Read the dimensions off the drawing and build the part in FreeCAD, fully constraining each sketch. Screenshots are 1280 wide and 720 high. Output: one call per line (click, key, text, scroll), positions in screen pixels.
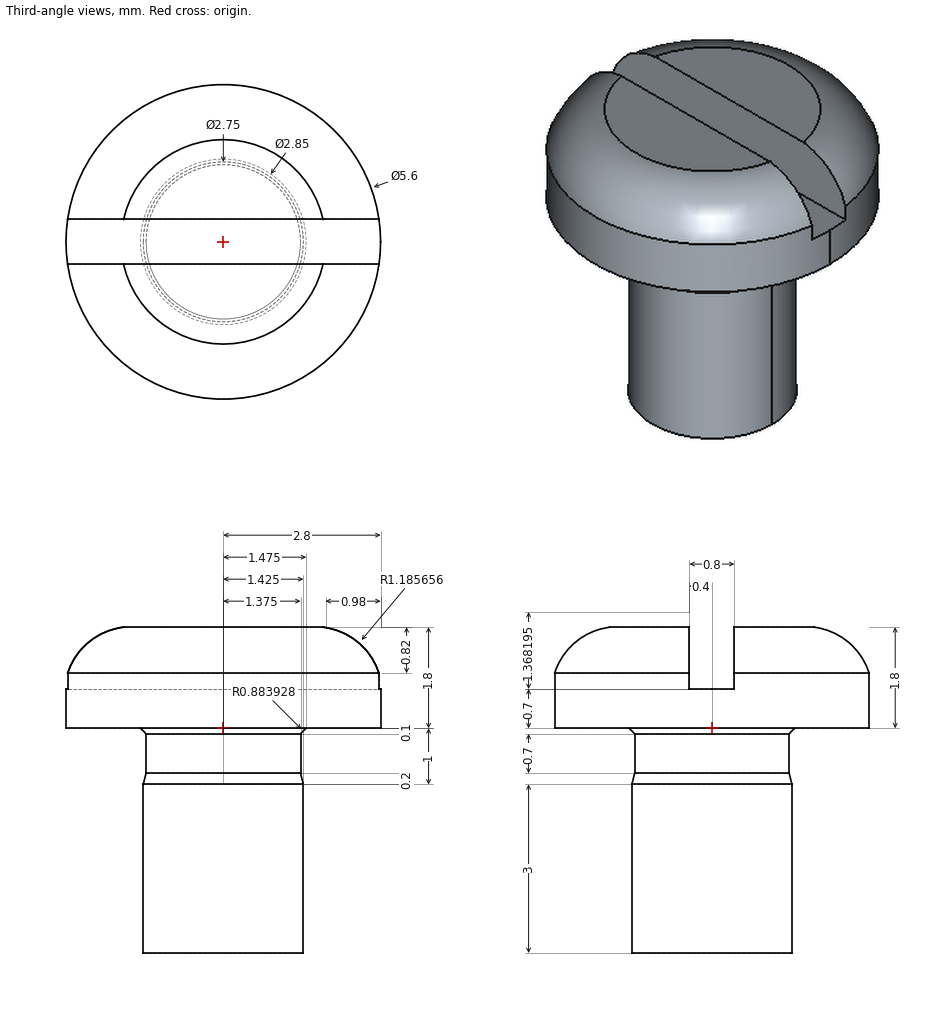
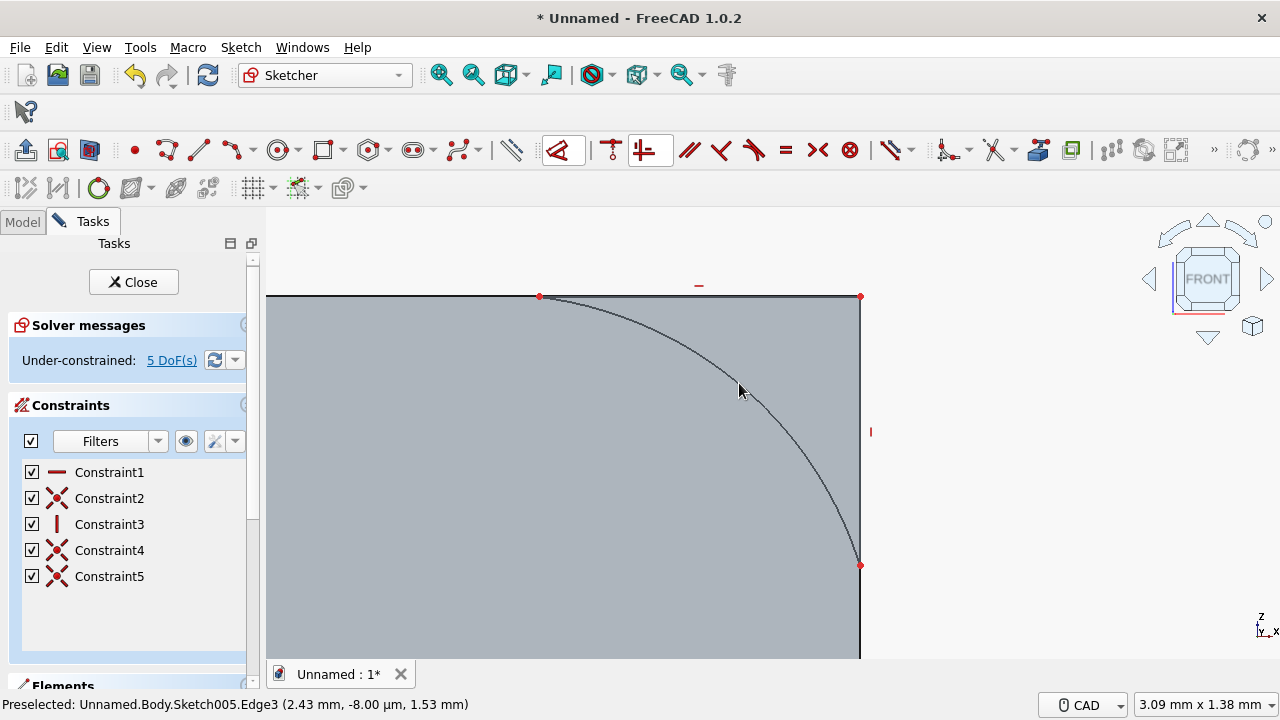
click(800, 448)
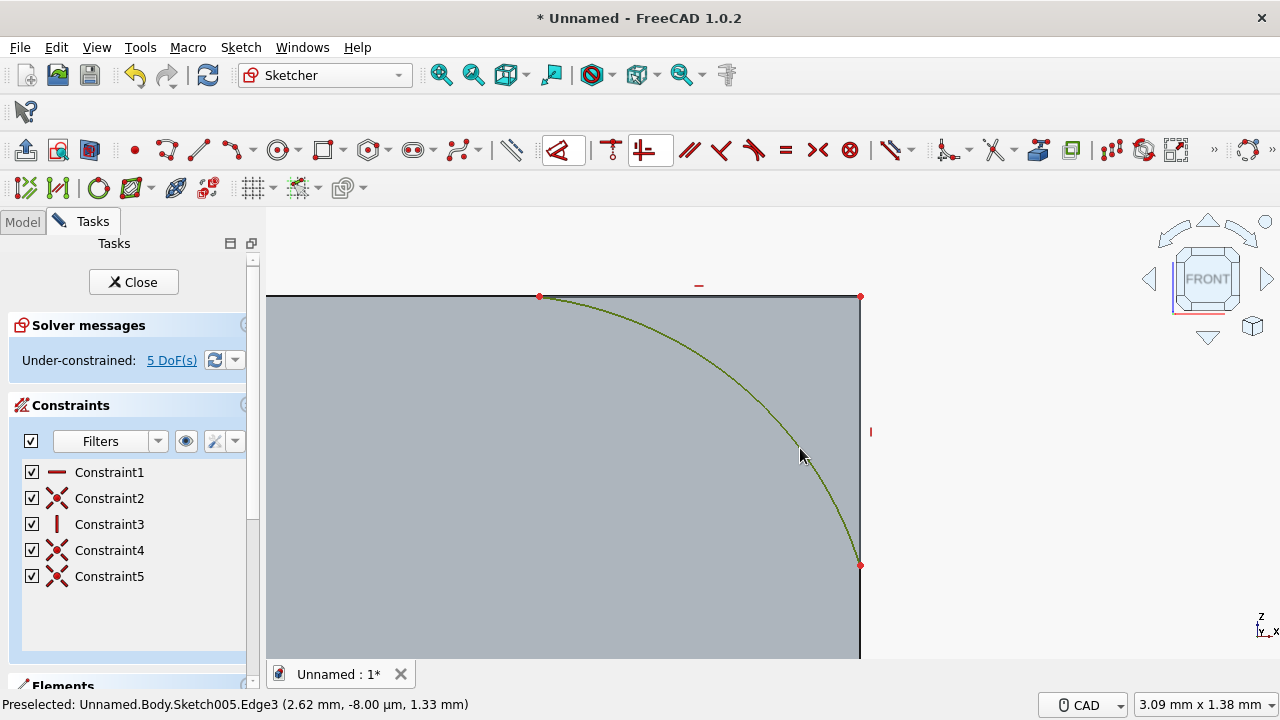
click(580, 150)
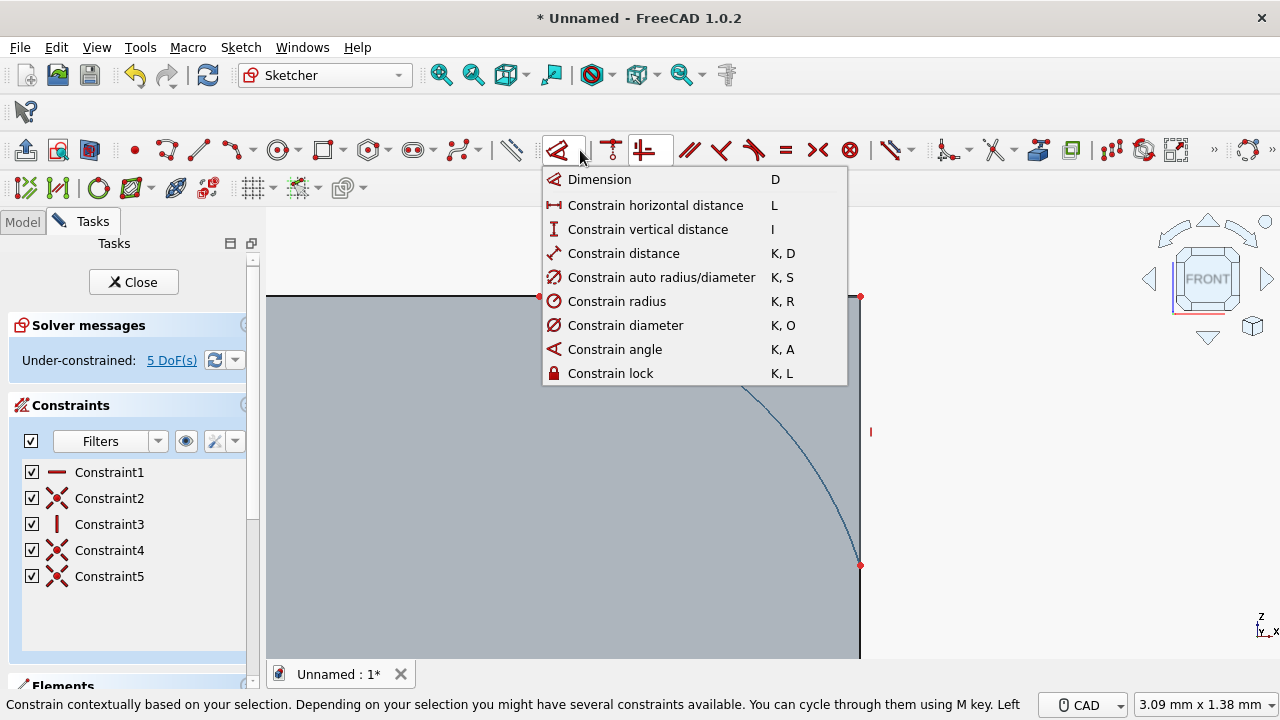
click(695, 301)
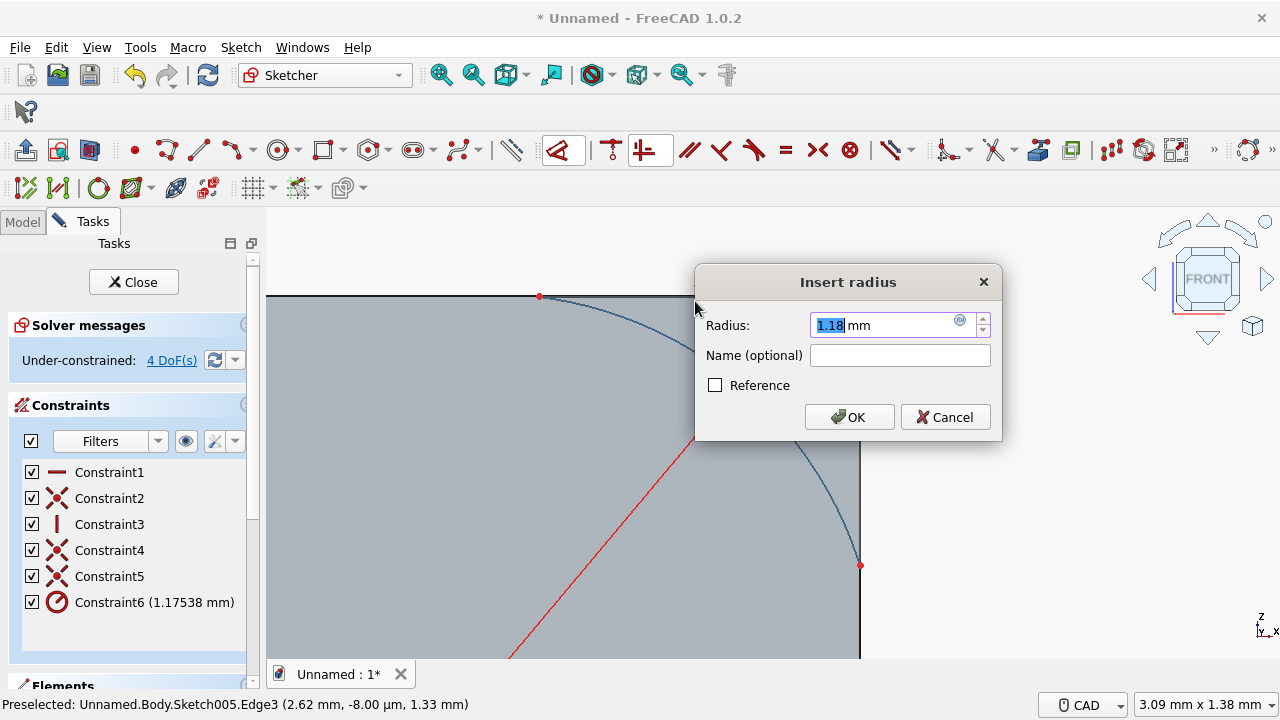
text(1.185656)
key(Return)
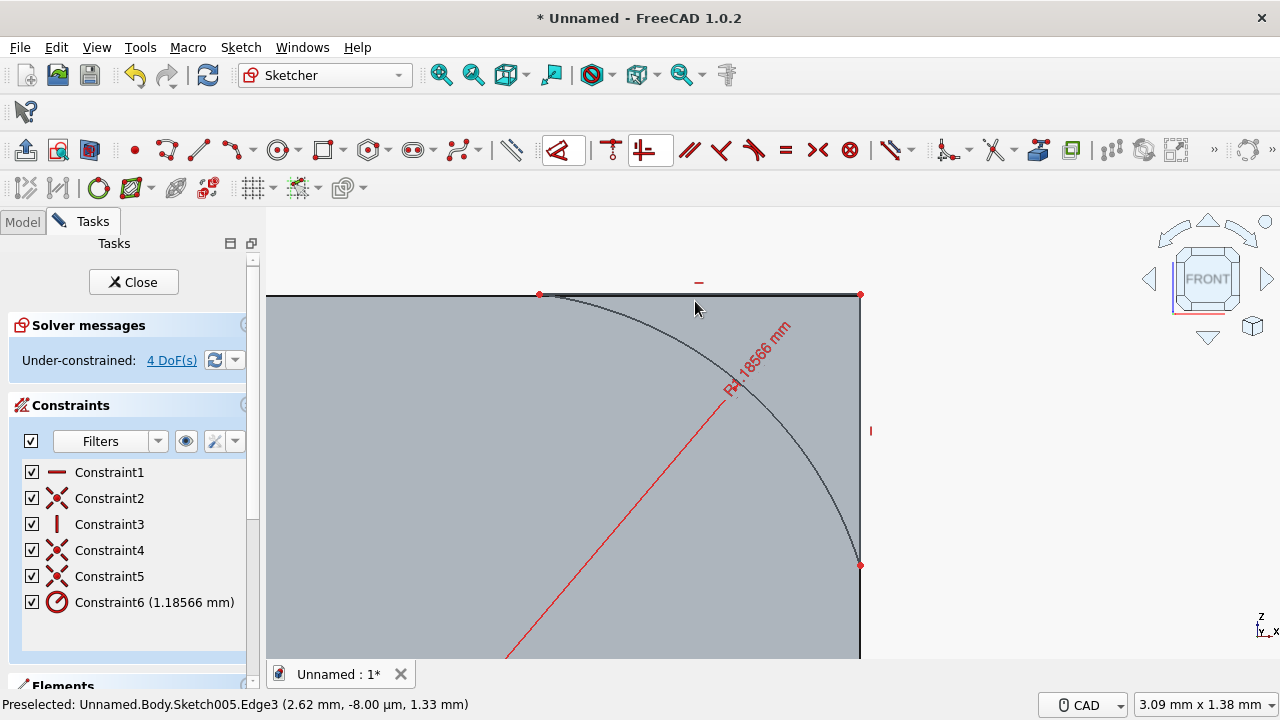
click(635, 294)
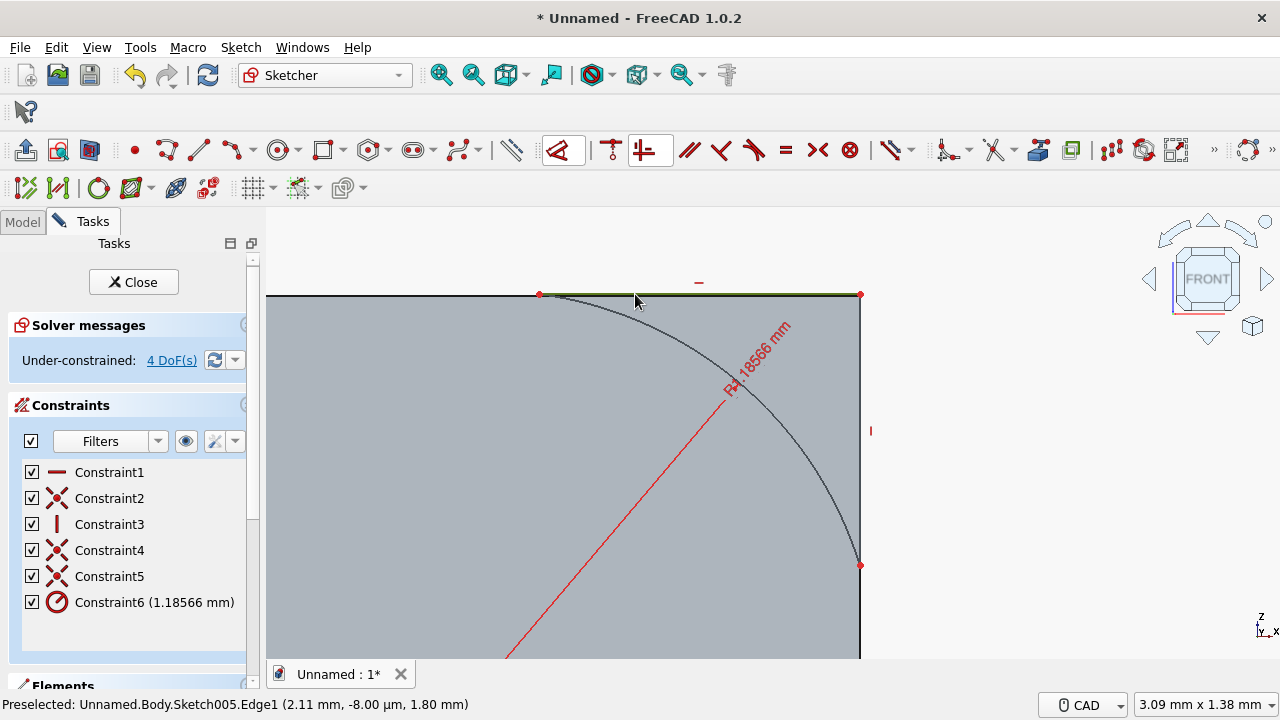
click(580, 150)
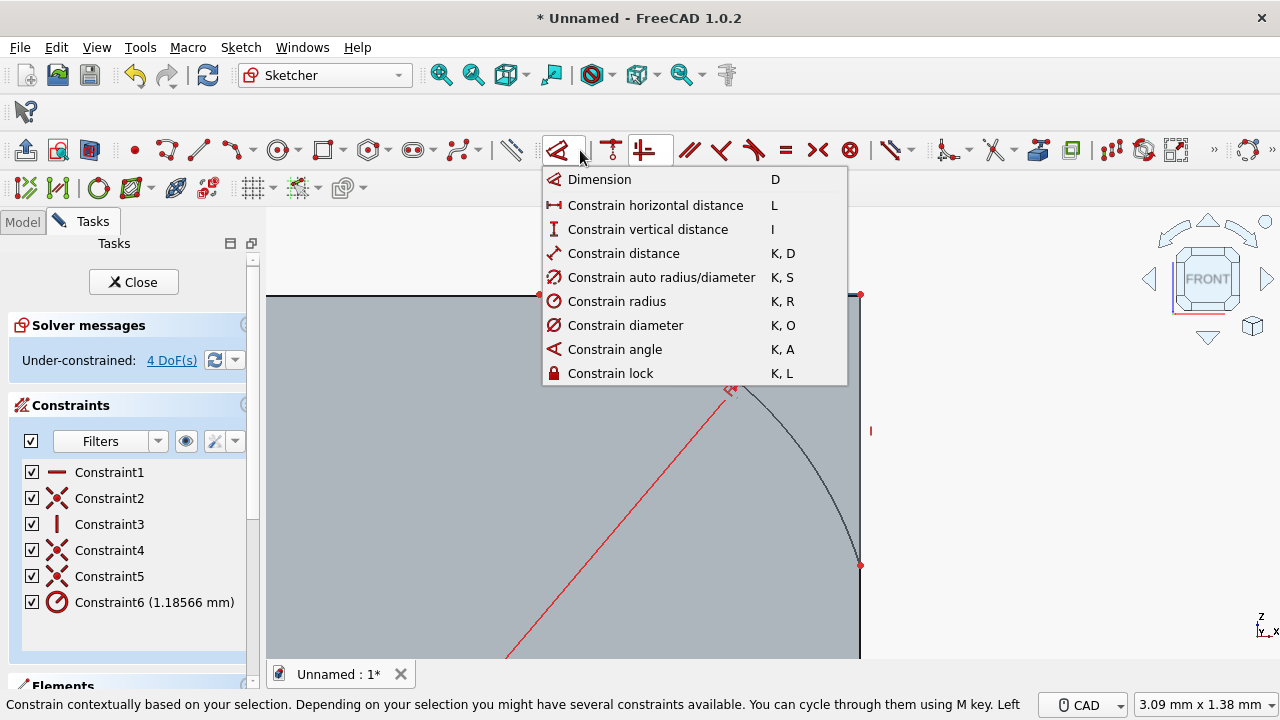
click(695, 205)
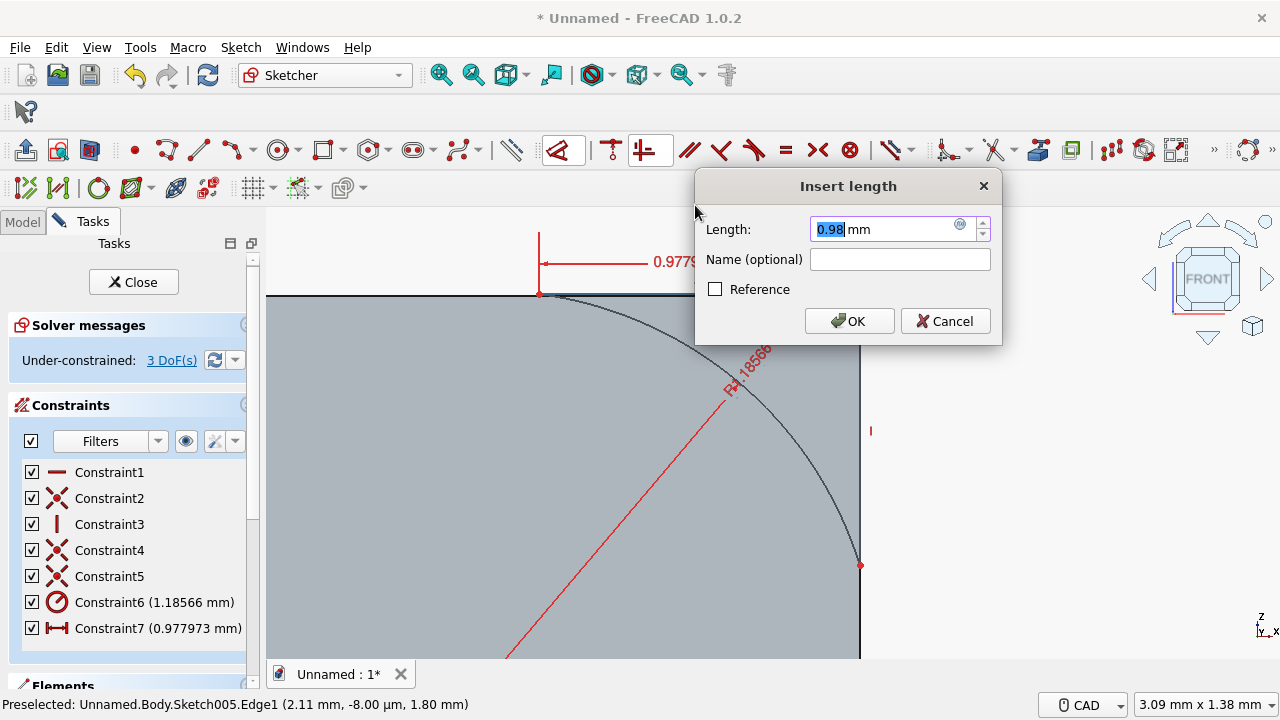
text(0.98)
key(Return)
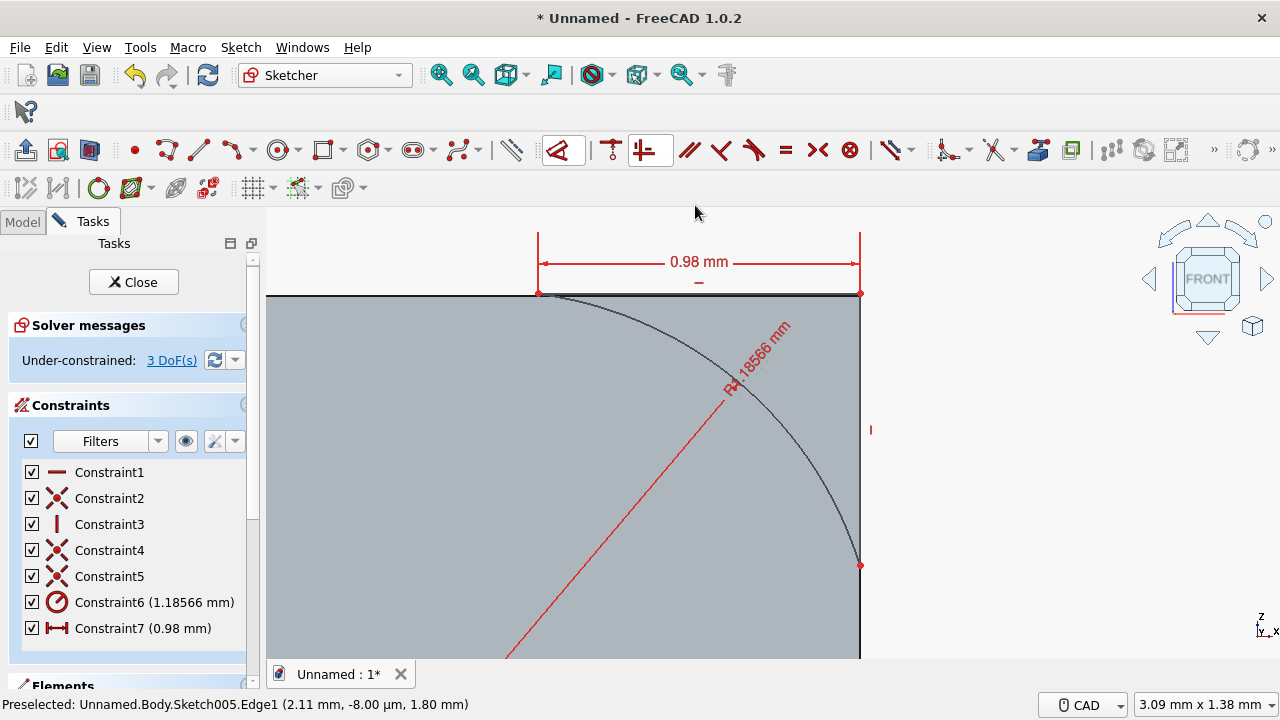
click(860, 376)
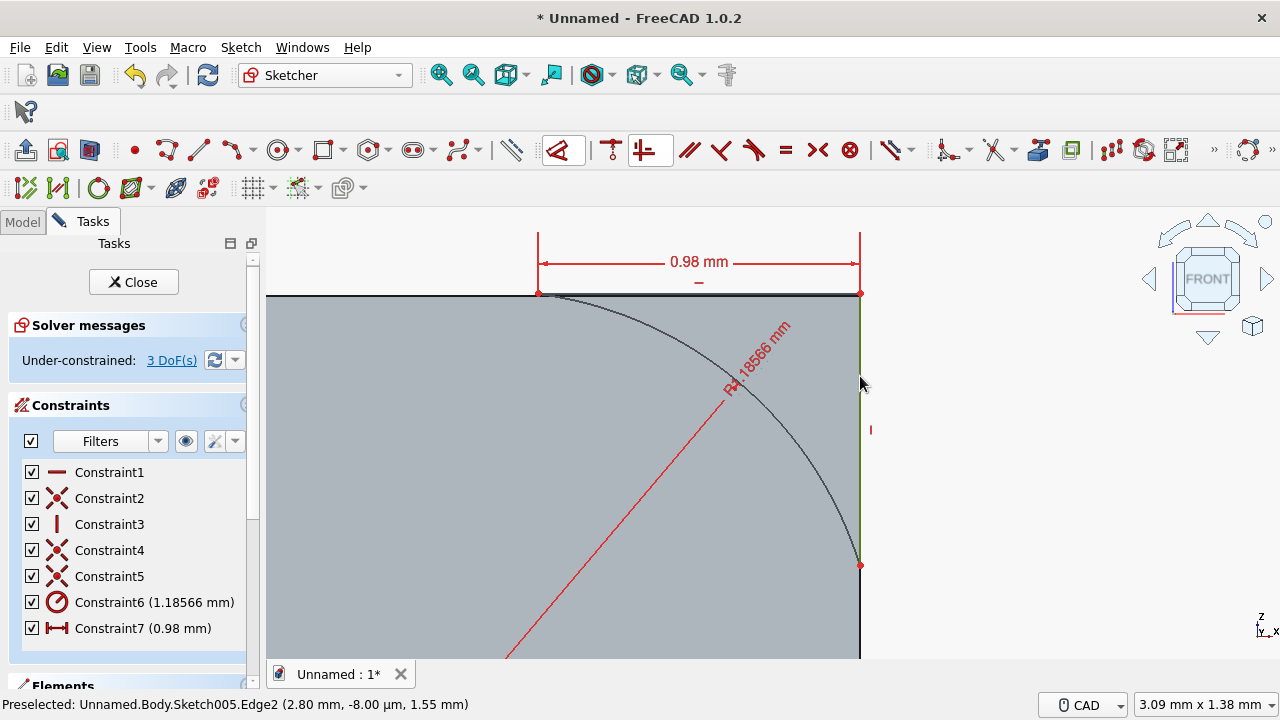
click(580, 150)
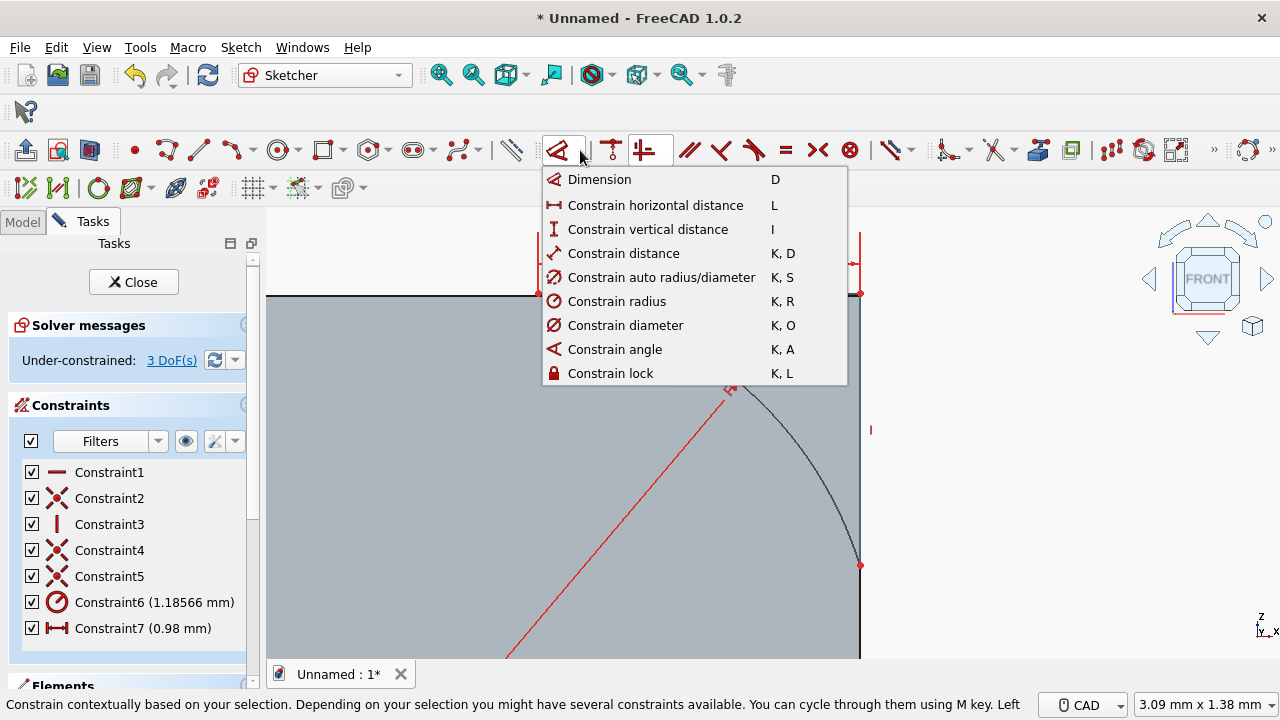
click(695, 229)